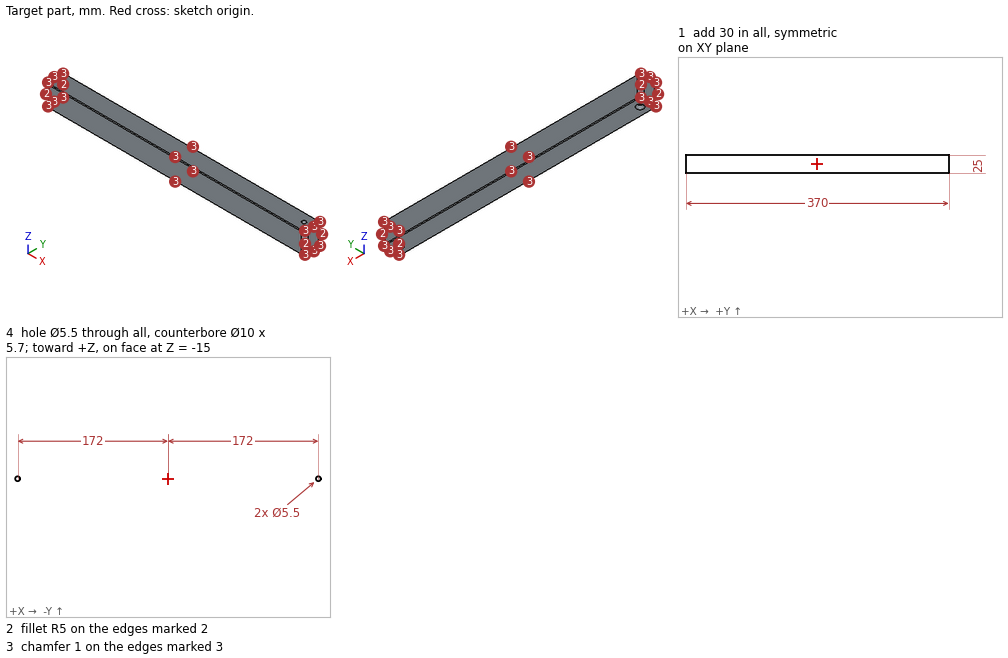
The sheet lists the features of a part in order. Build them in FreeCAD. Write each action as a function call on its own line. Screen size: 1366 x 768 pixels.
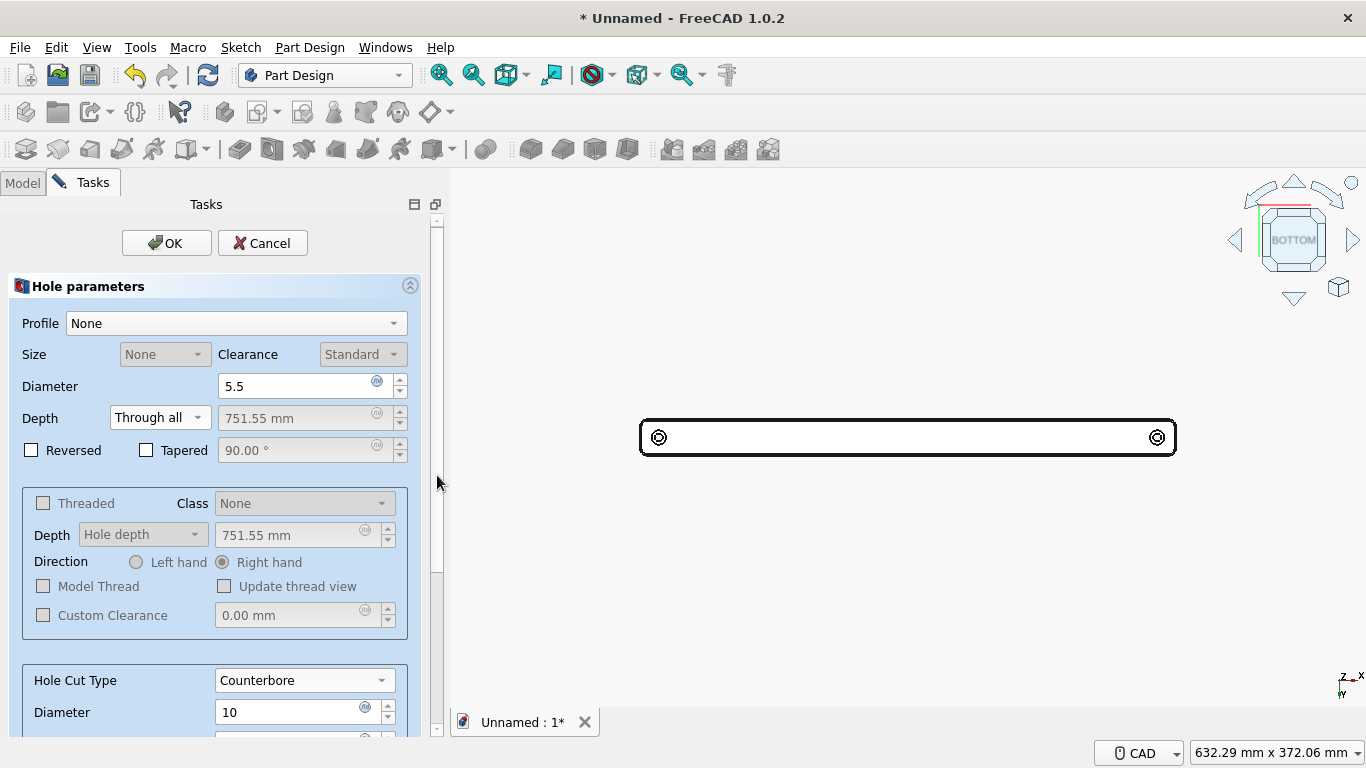
click(167, 243)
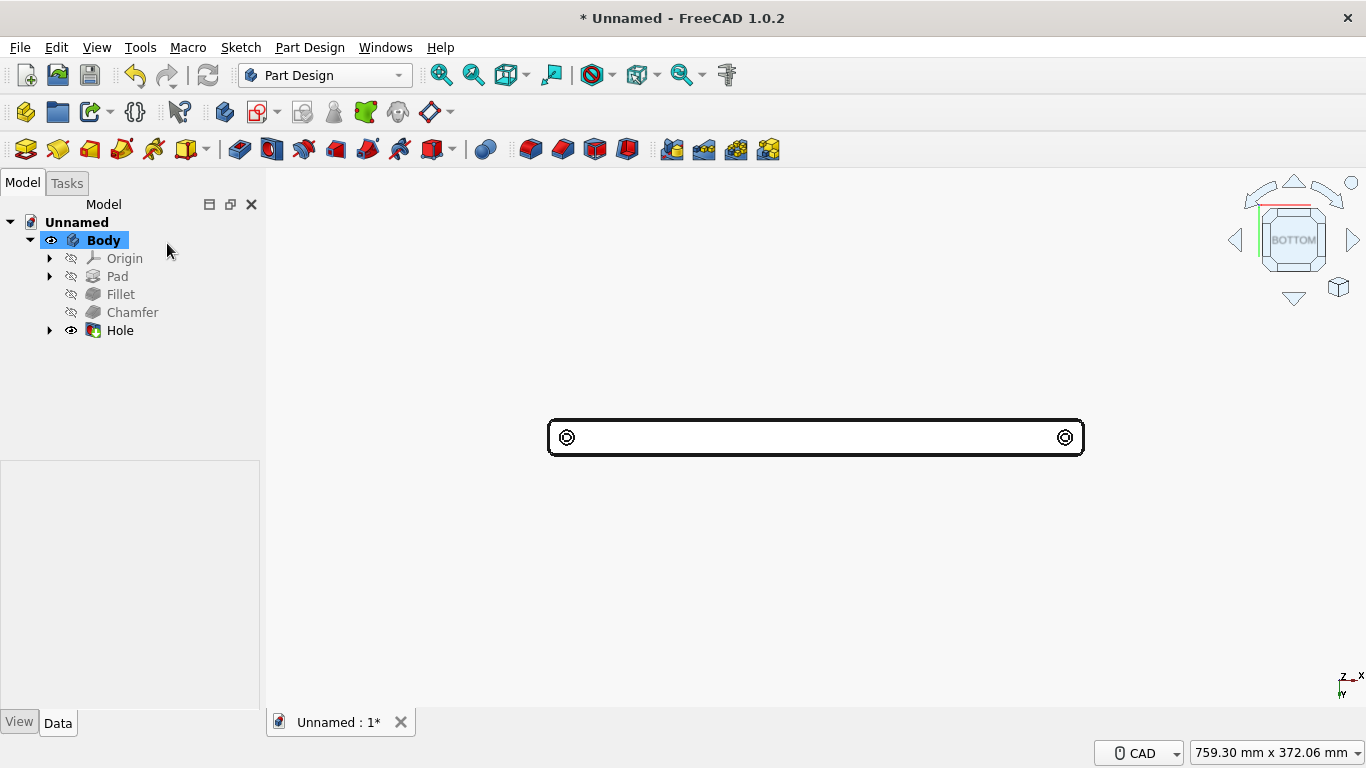
key(0)